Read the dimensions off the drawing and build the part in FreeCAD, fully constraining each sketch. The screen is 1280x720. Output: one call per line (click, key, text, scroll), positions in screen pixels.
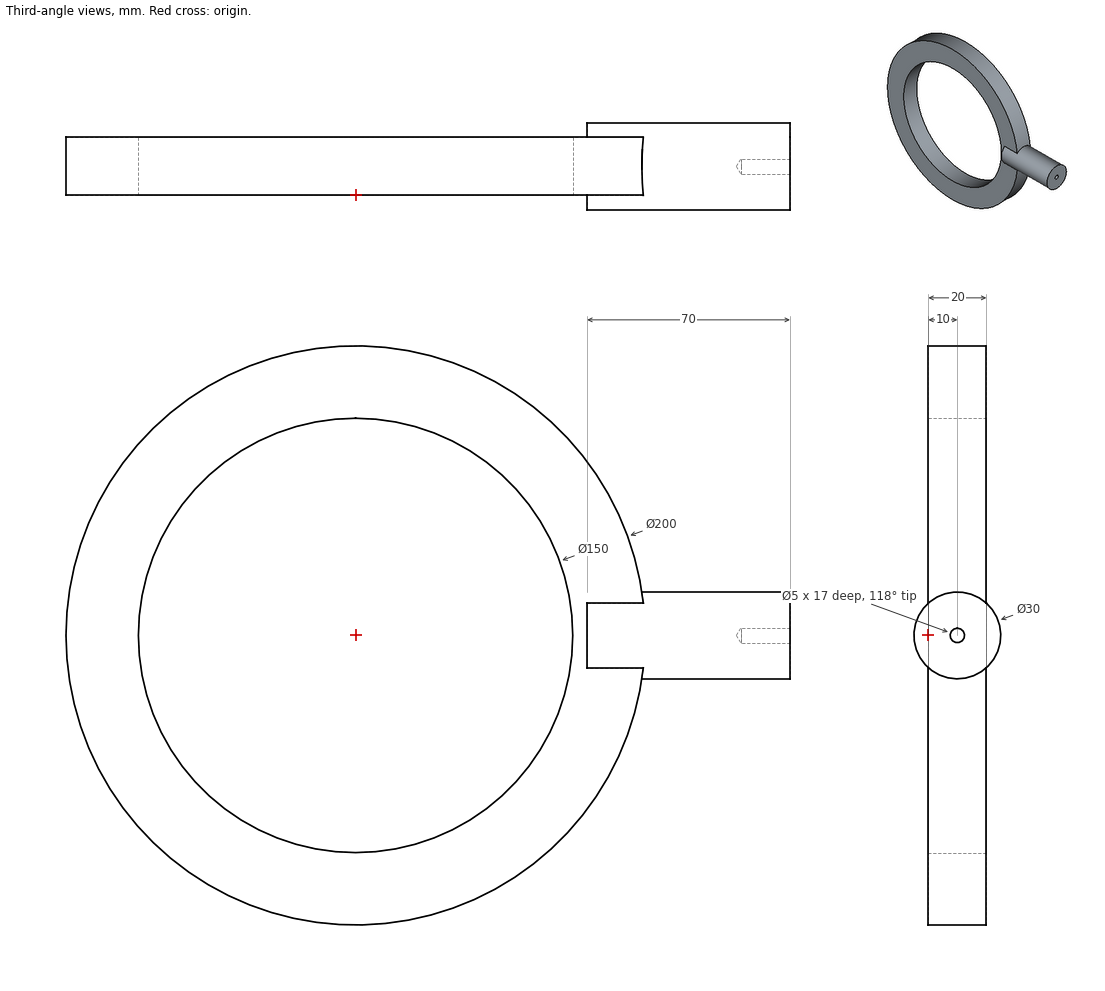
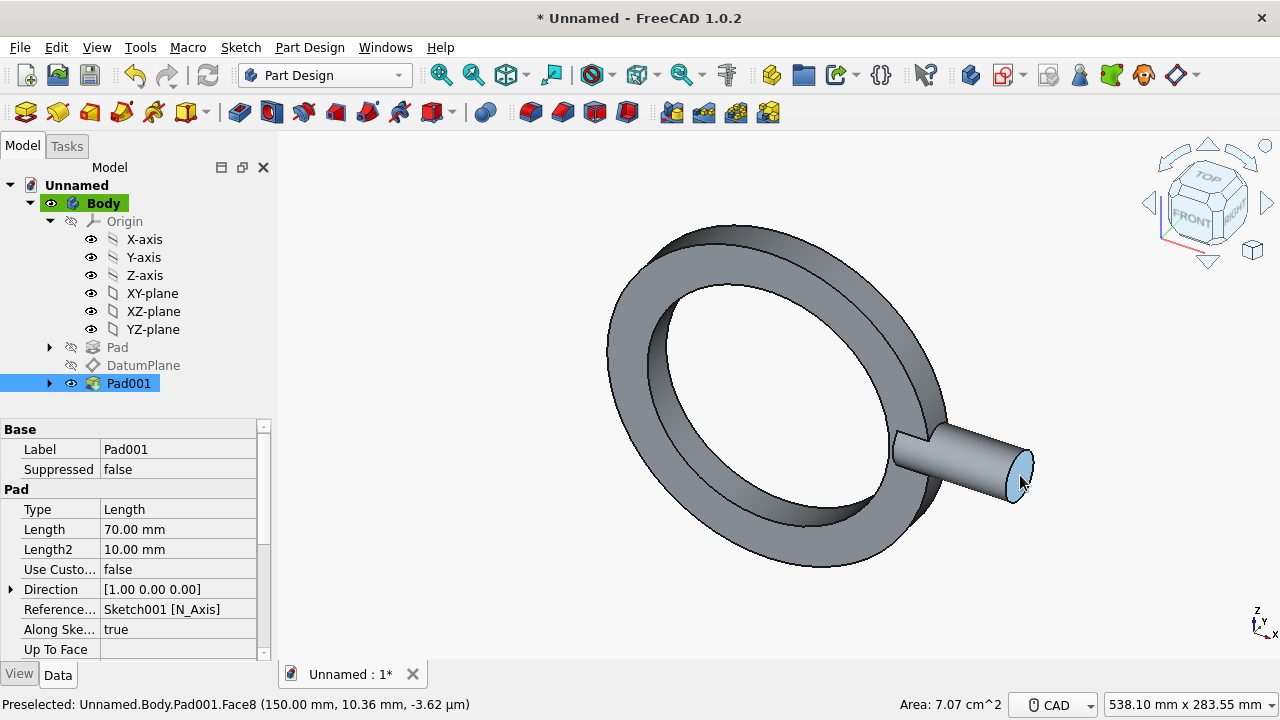
click(1004, 76)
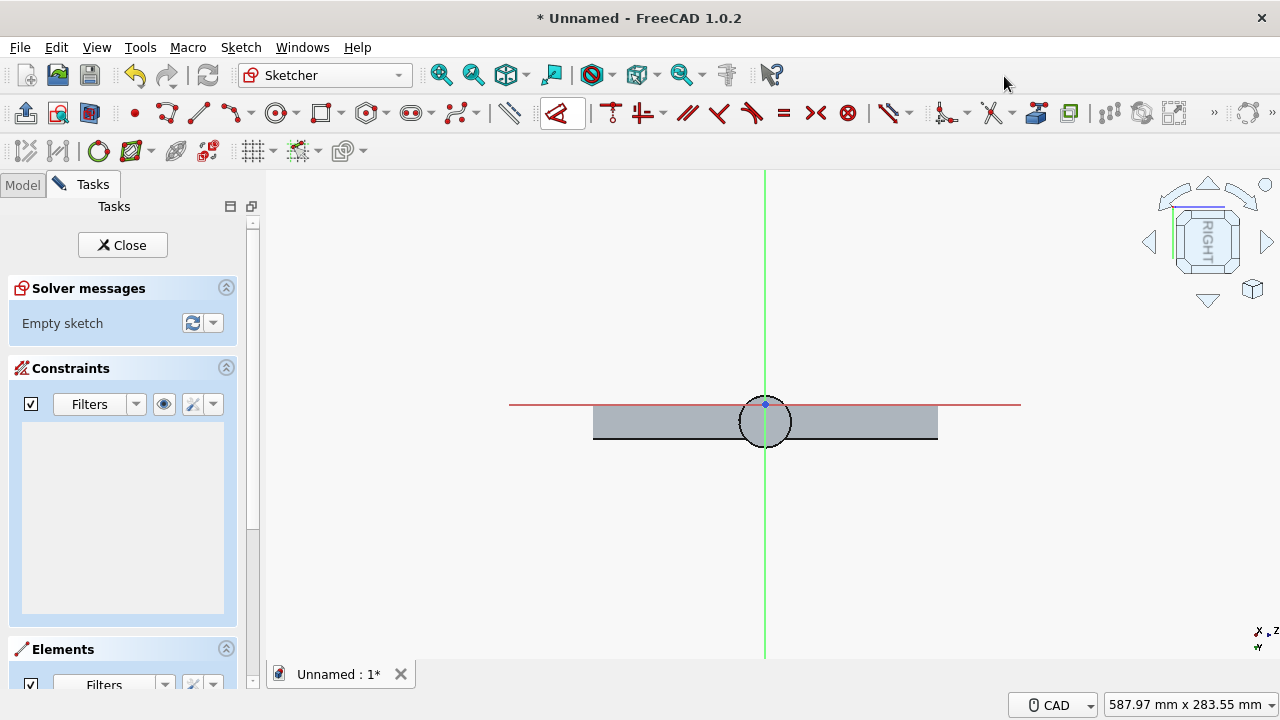
scroll(768, 422, up, 15)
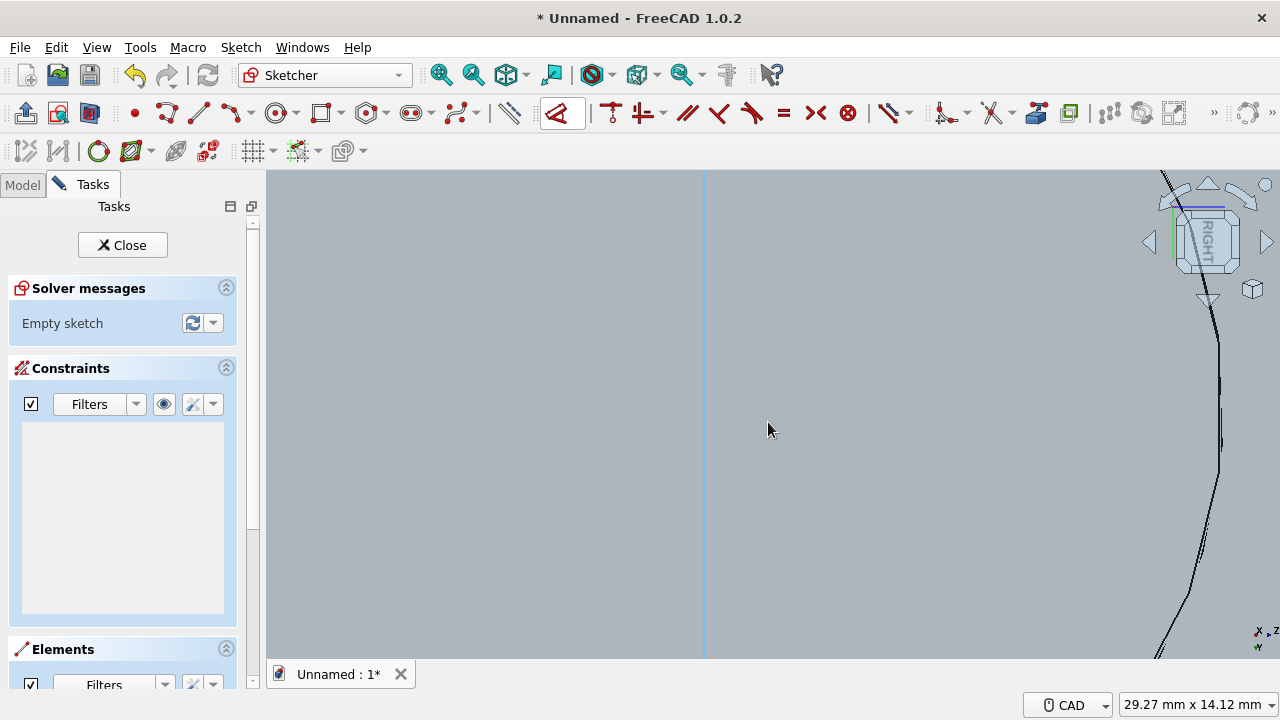
scroll(702, 400, up, 3)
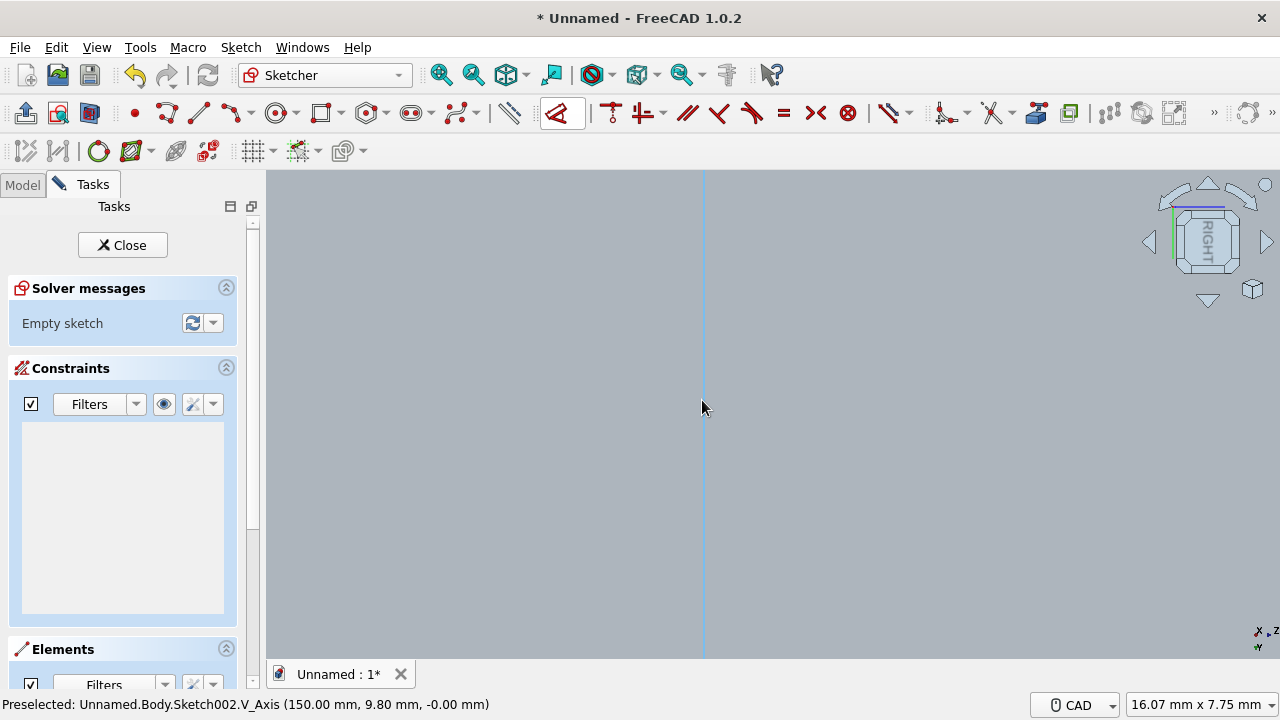
key(g)
key(c)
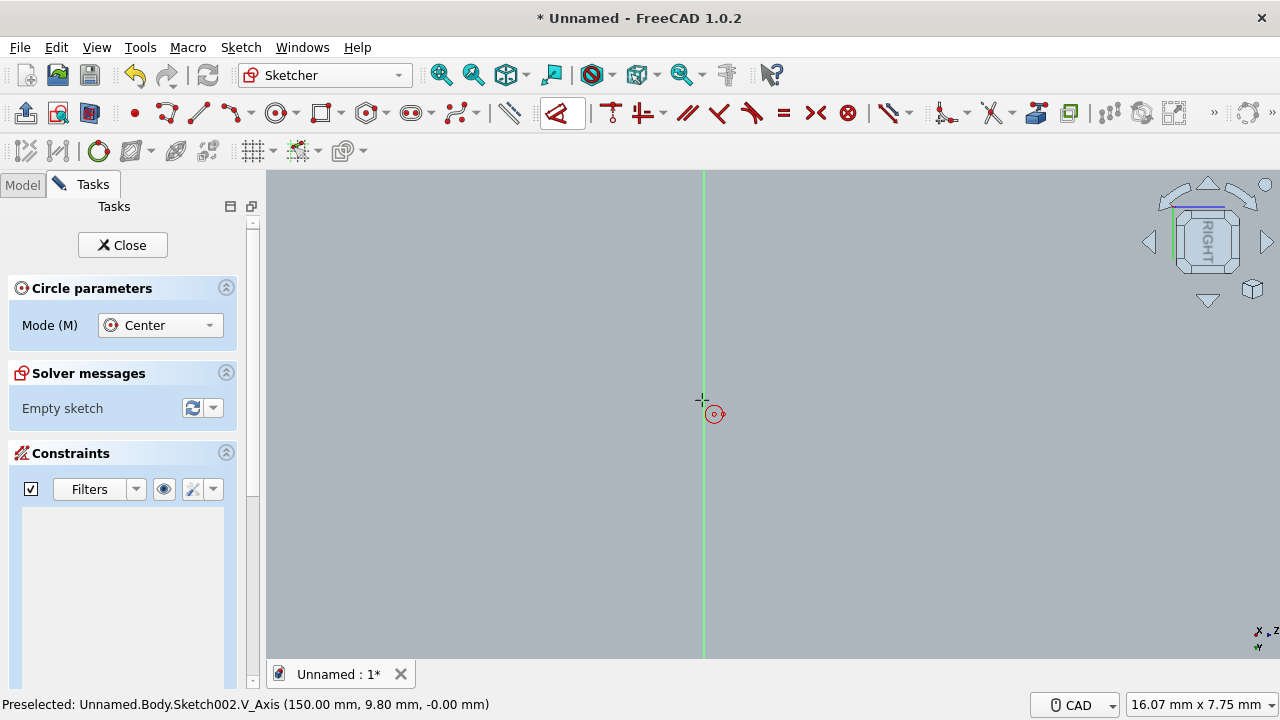
click(704, 414)
click(816, 302)
key(Escape)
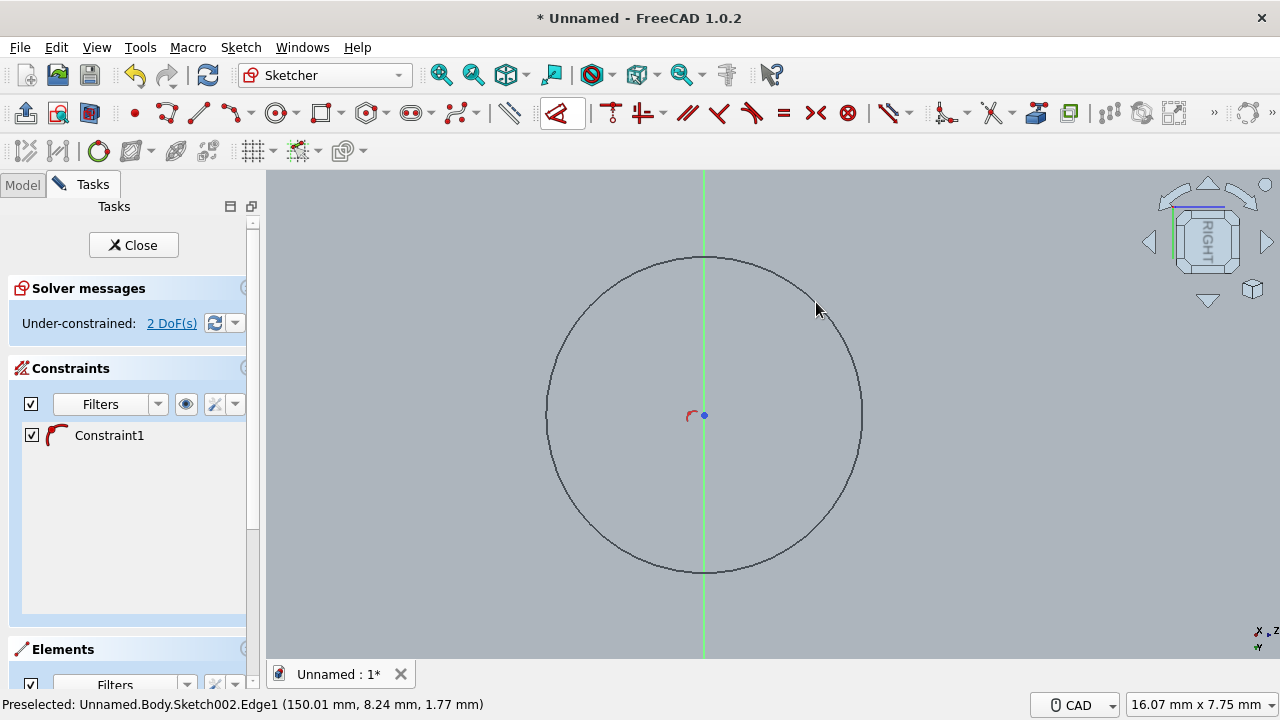
click(556, 114)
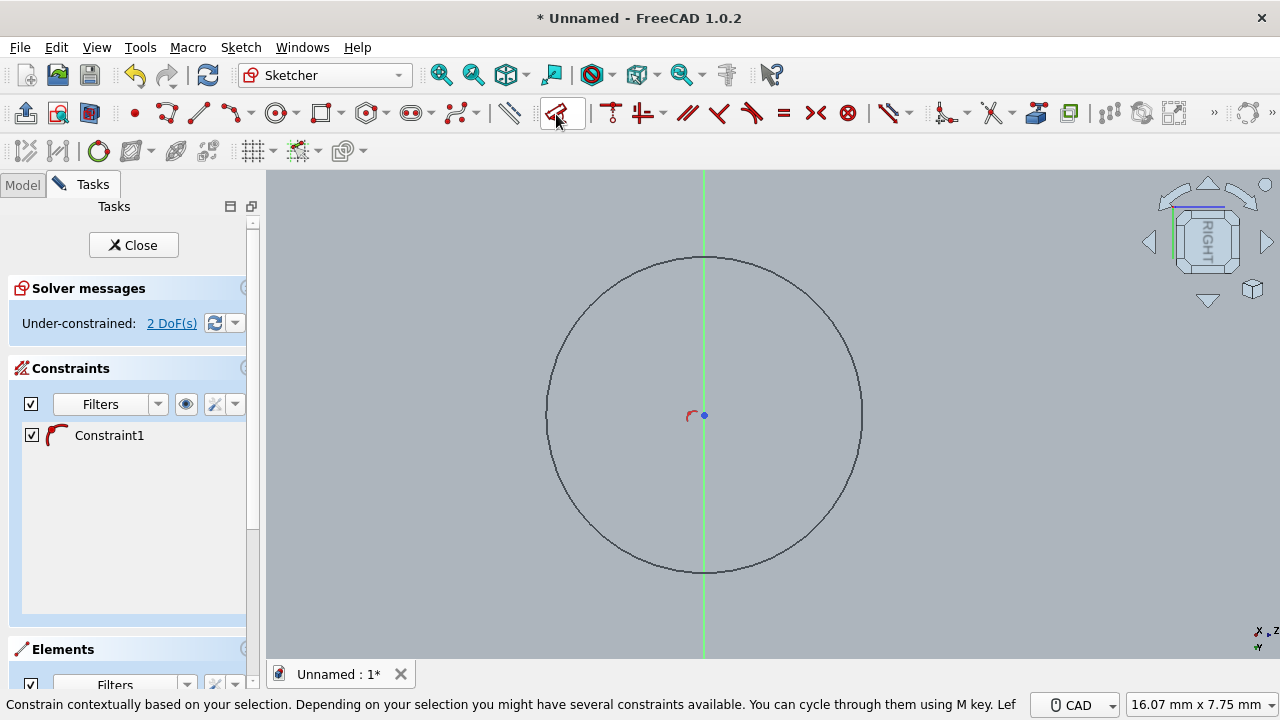
click(816, 303)
click(839, 280)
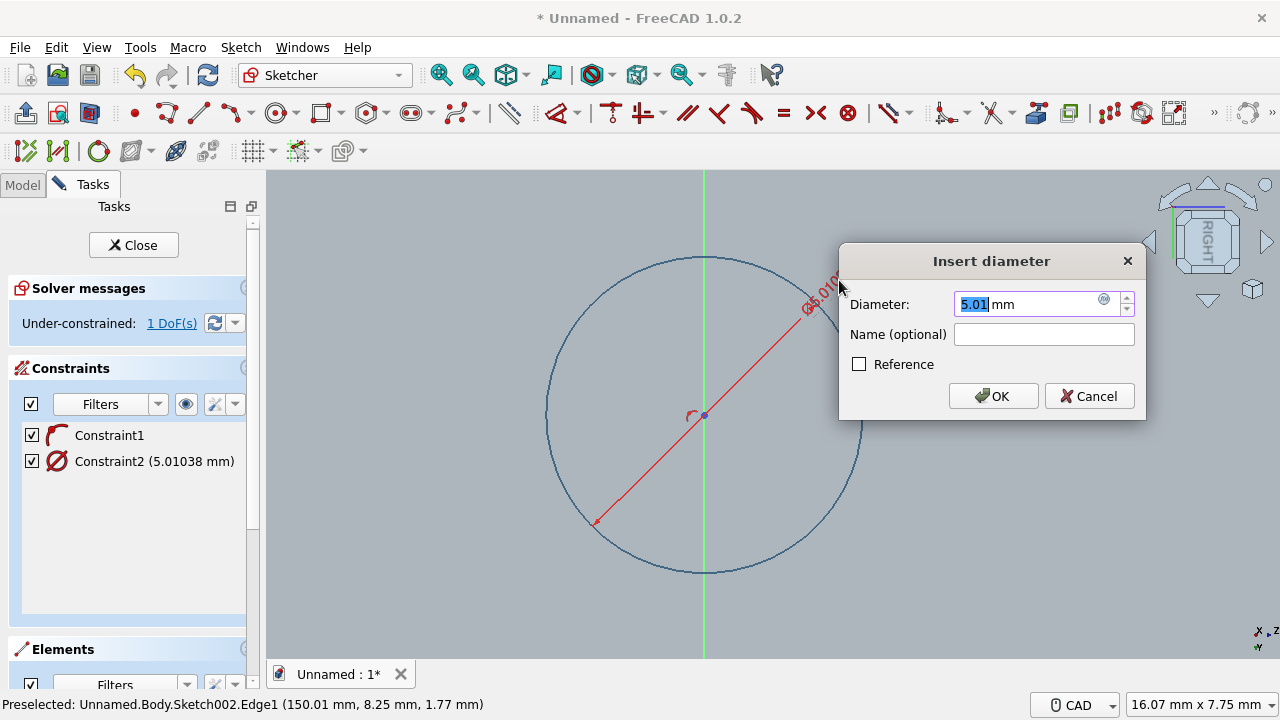
text(5)
key(Return)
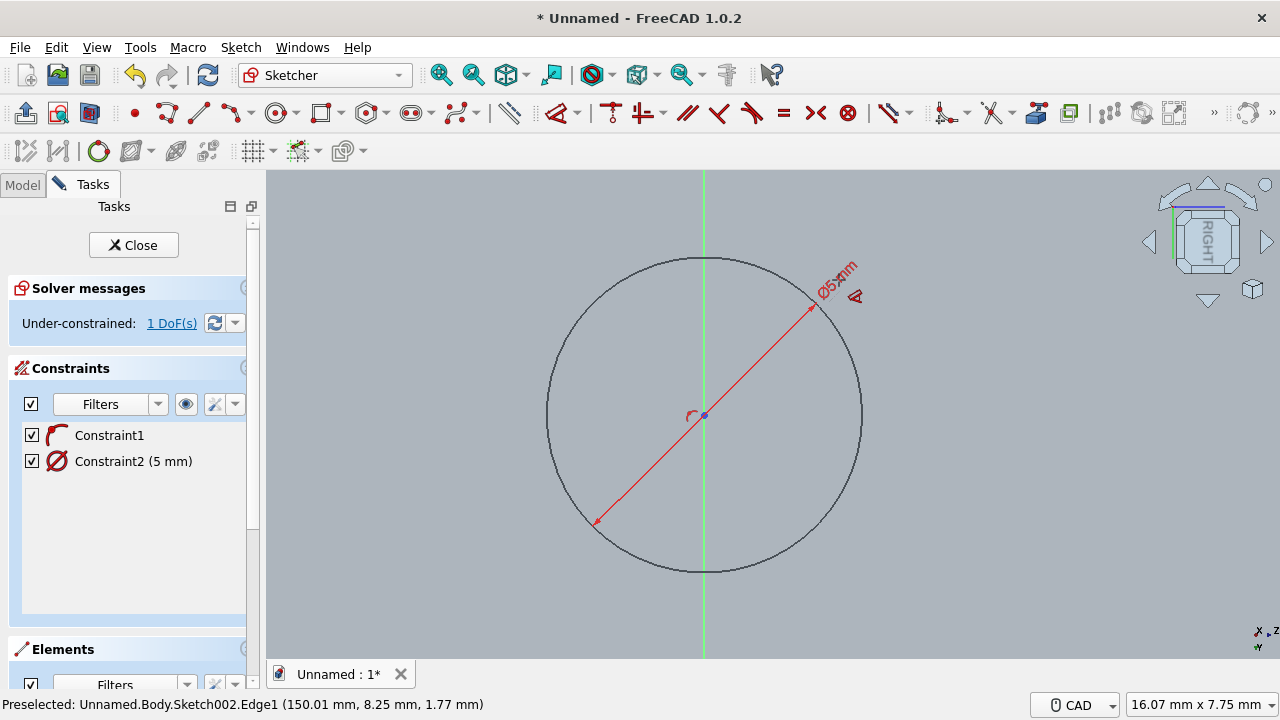
click(704, 415)
click(738, 306)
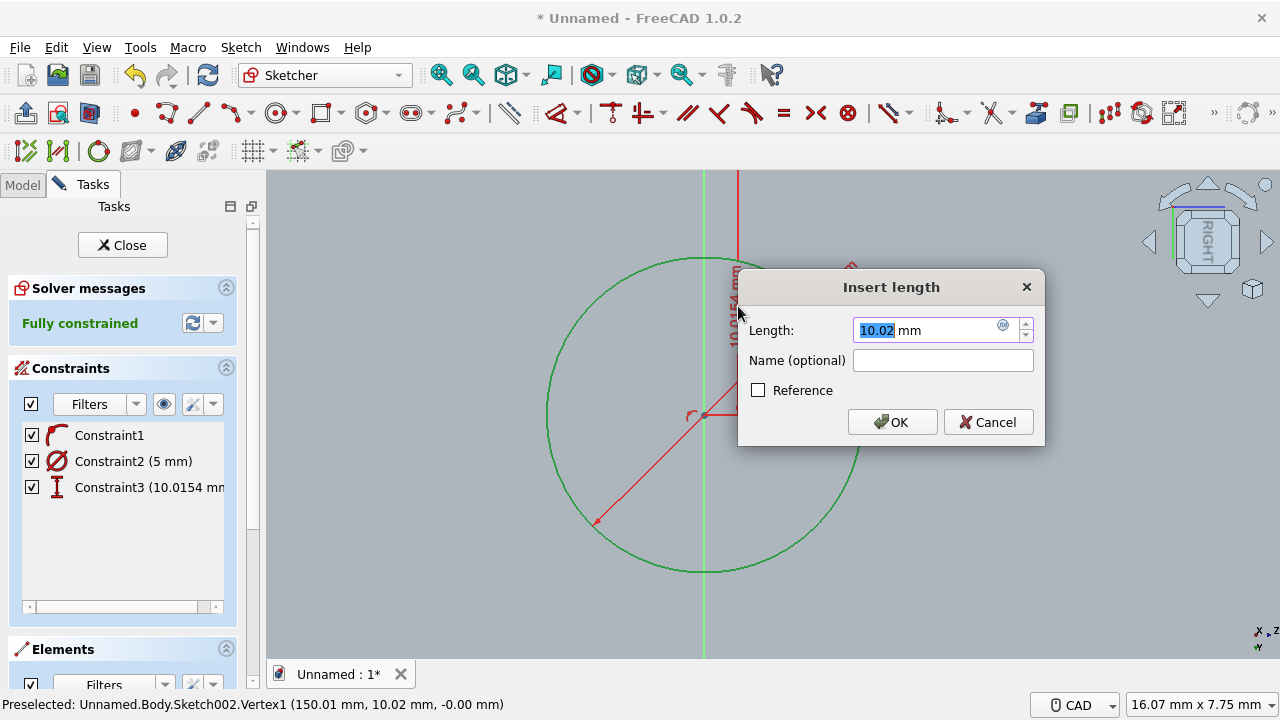
text(10)
key(Return)
key(Escape)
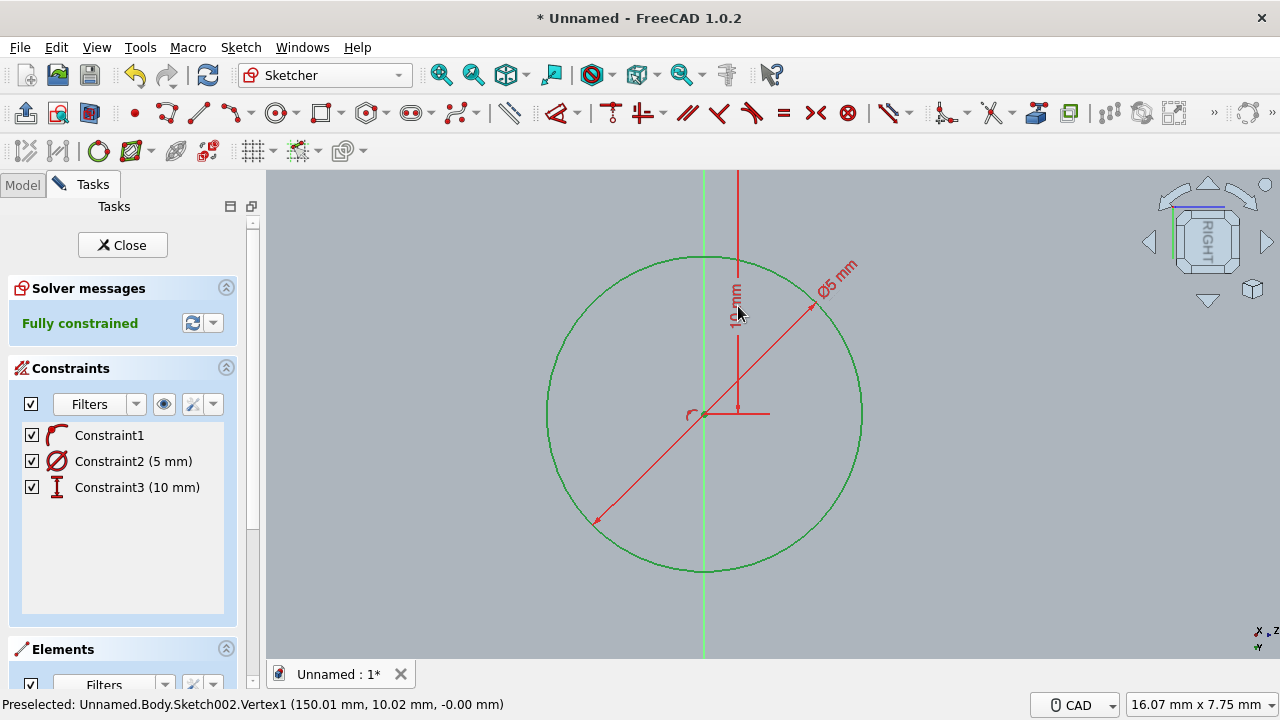
click(123, 245)